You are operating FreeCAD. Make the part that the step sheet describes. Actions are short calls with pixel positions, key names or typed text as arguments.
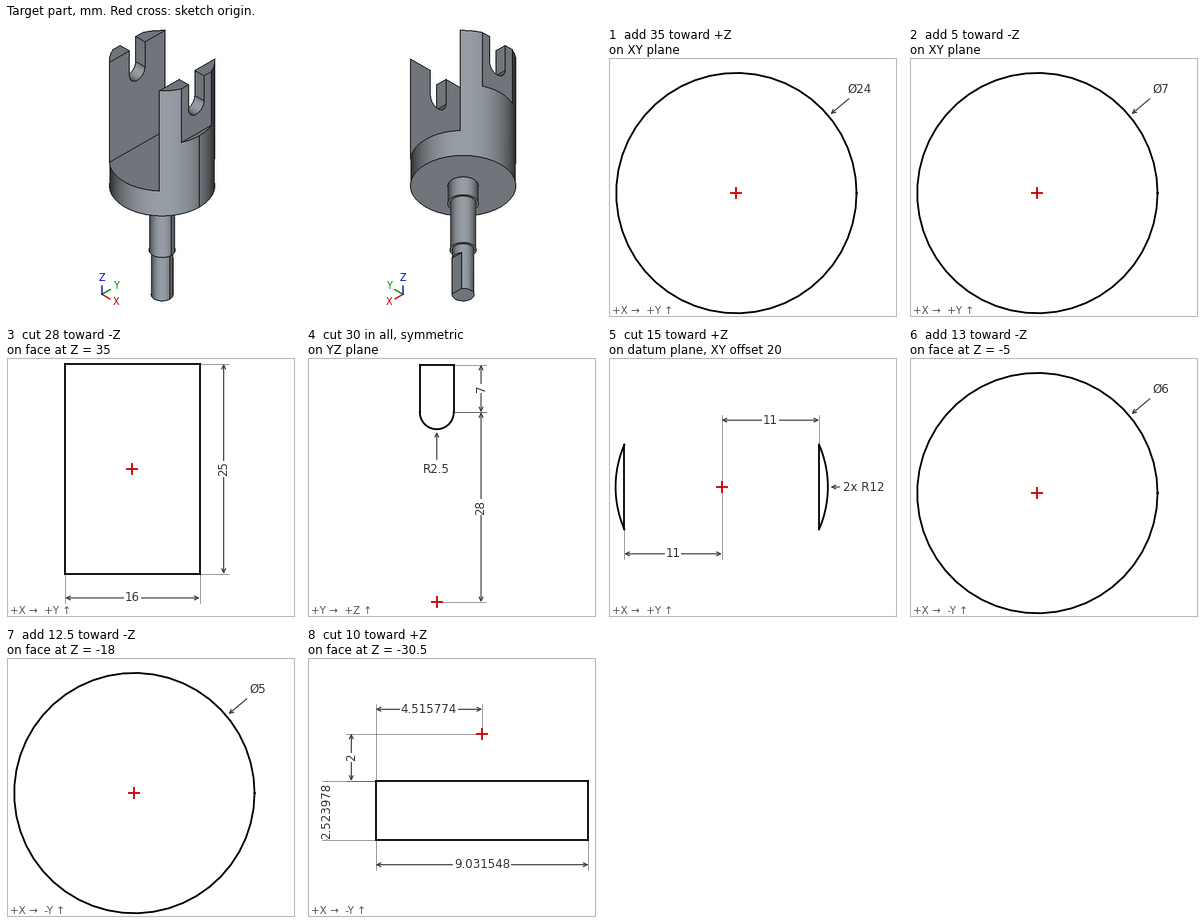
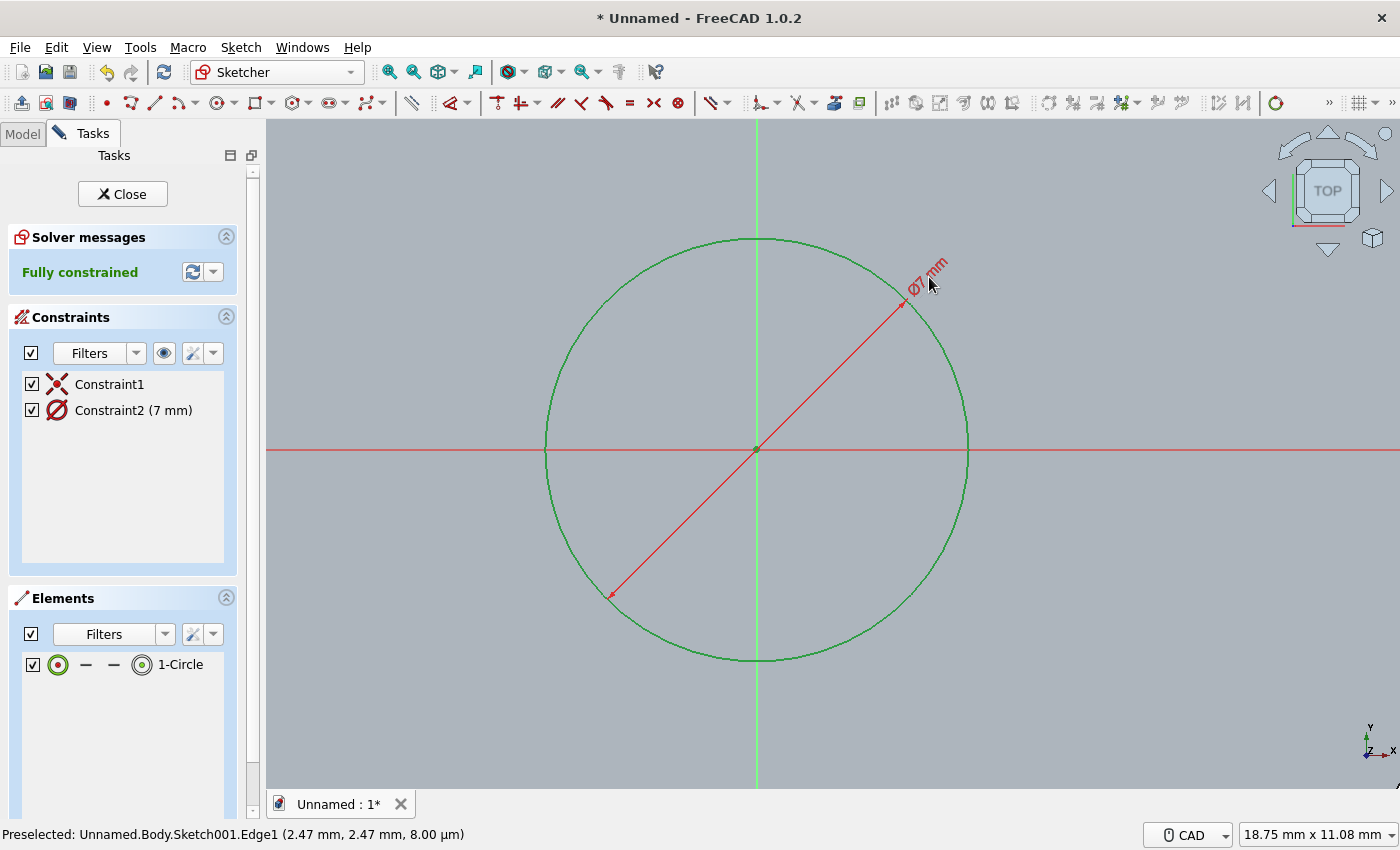
click(123, 194)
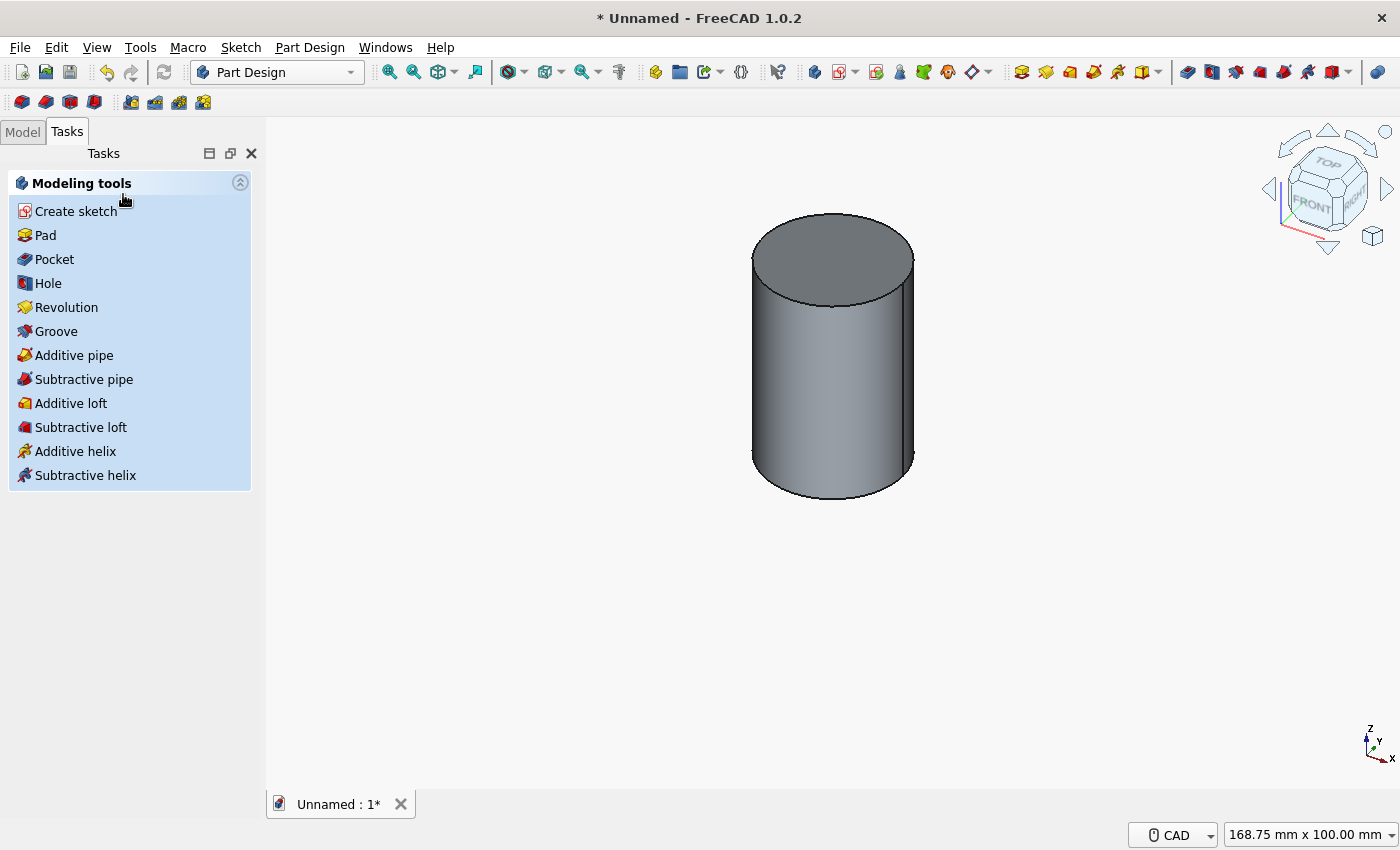
click(1022, 72)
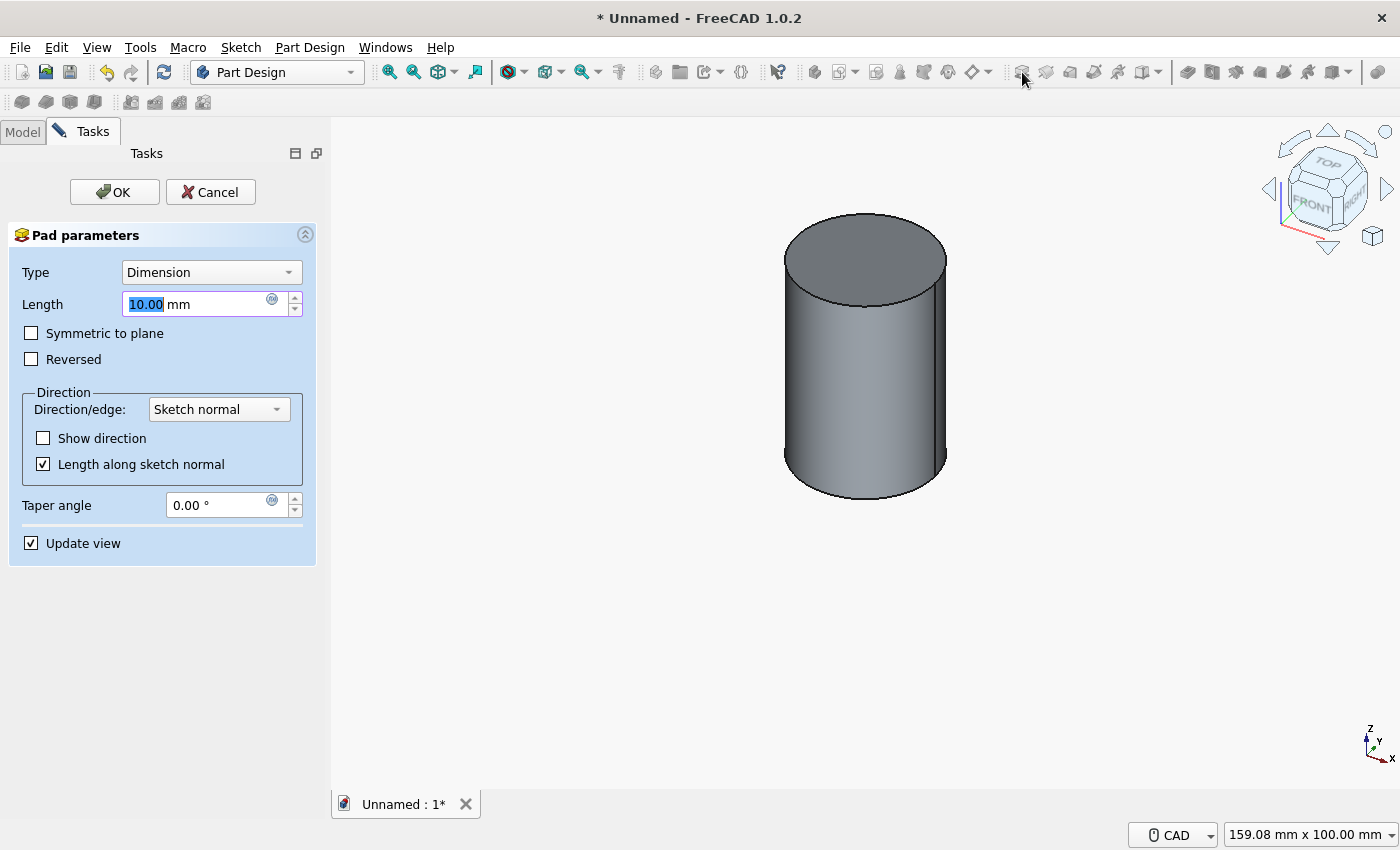
text(5)
key(Tab)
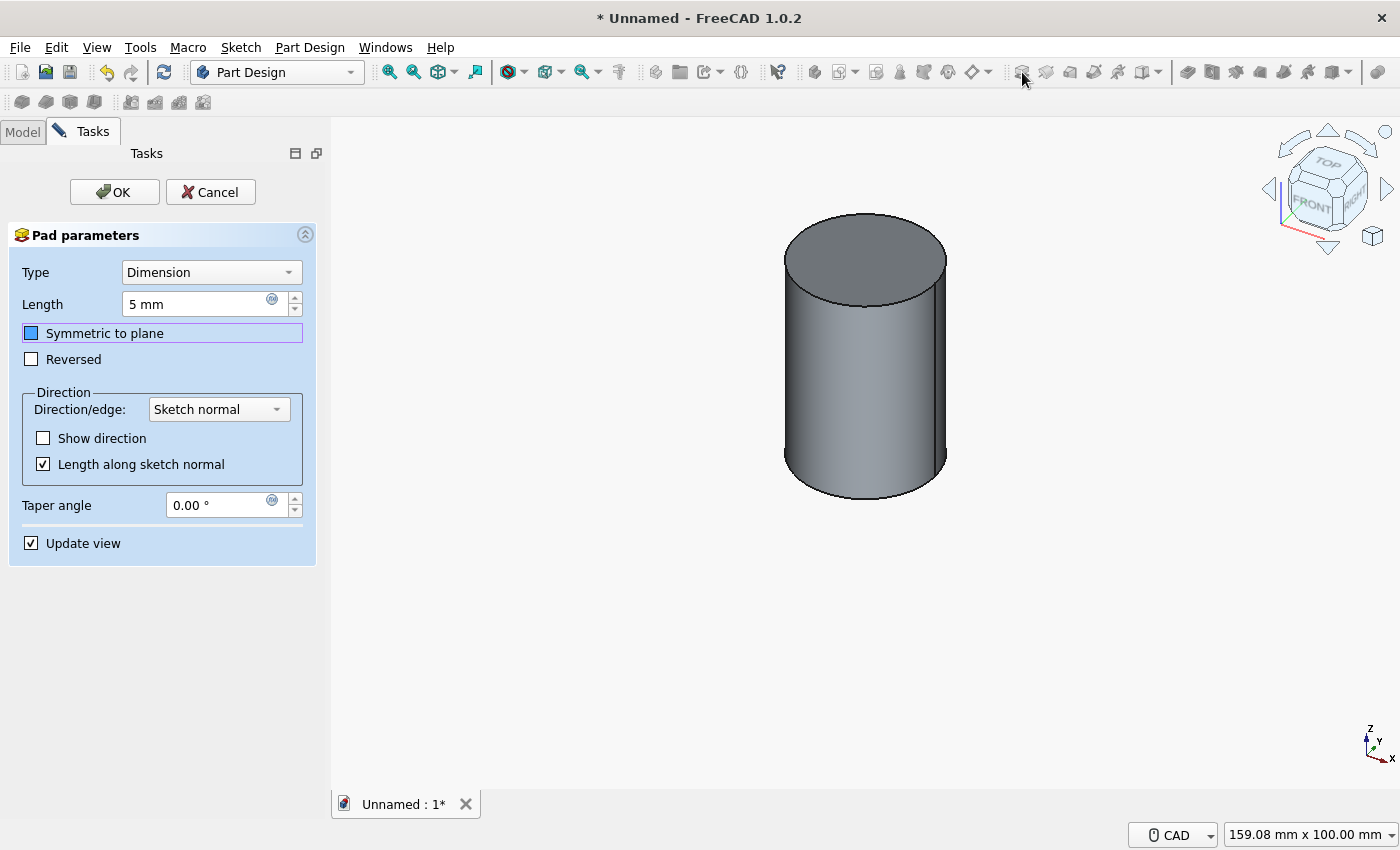
click(30, 359)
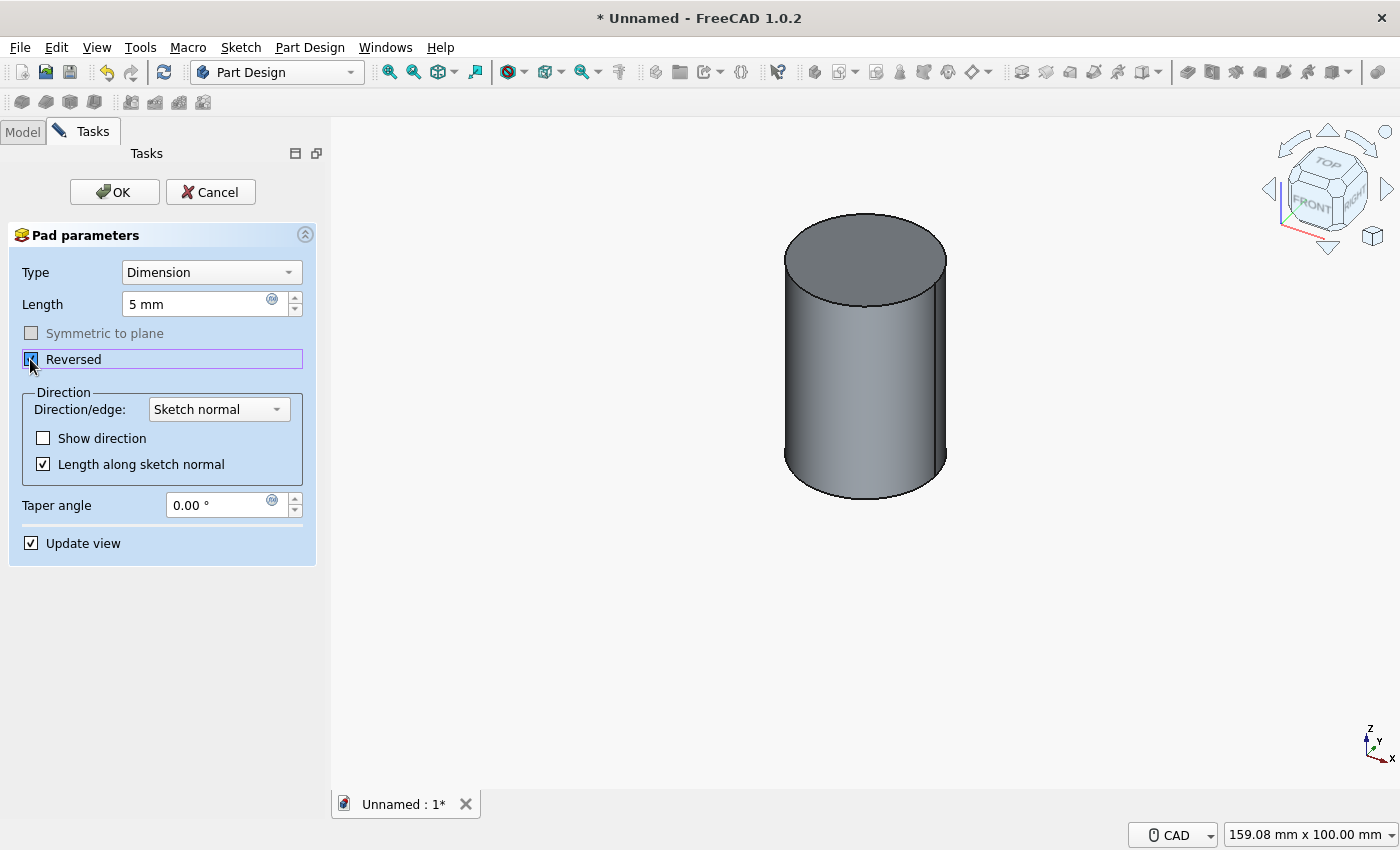
click(115, 192)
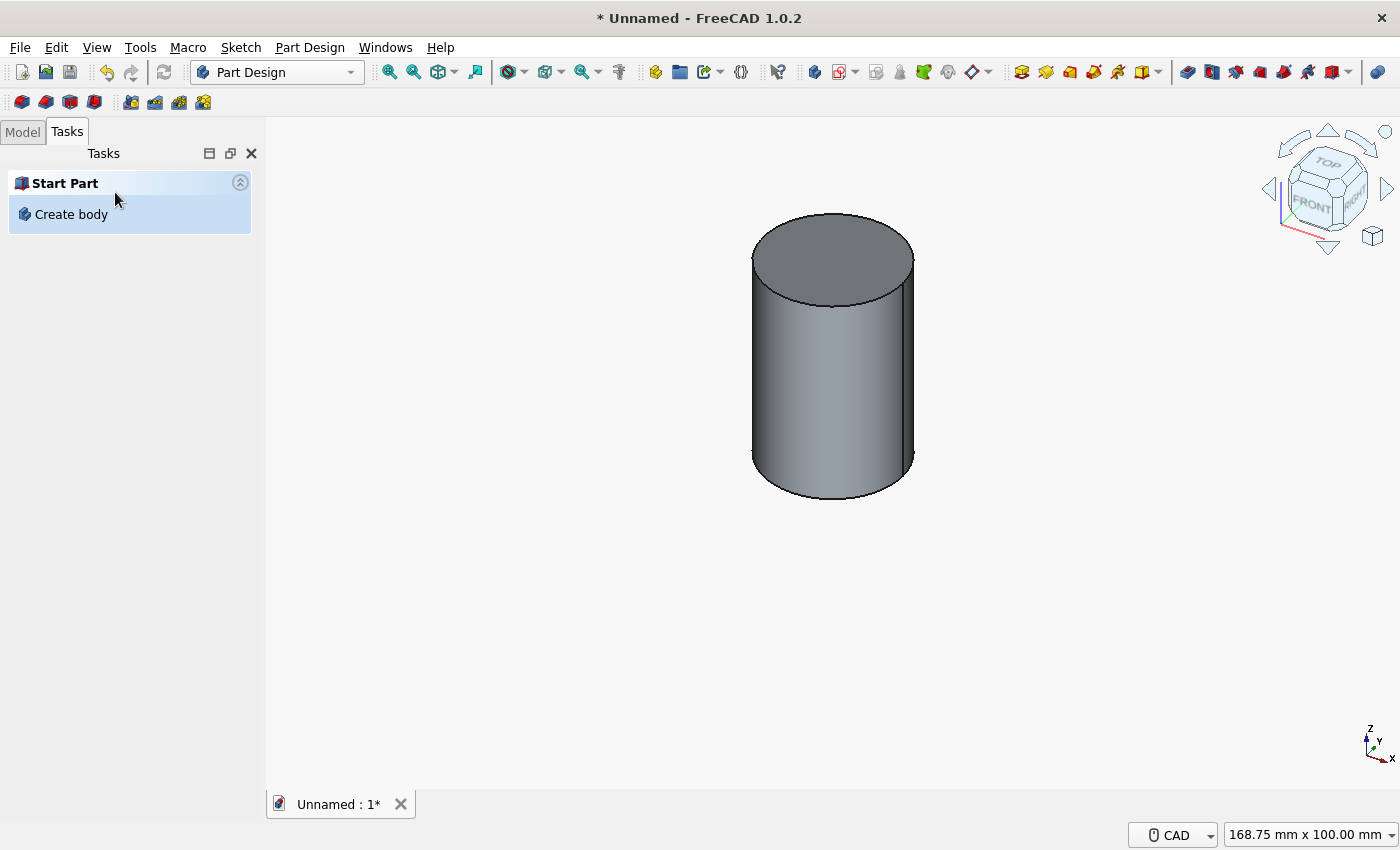
click(833, 259)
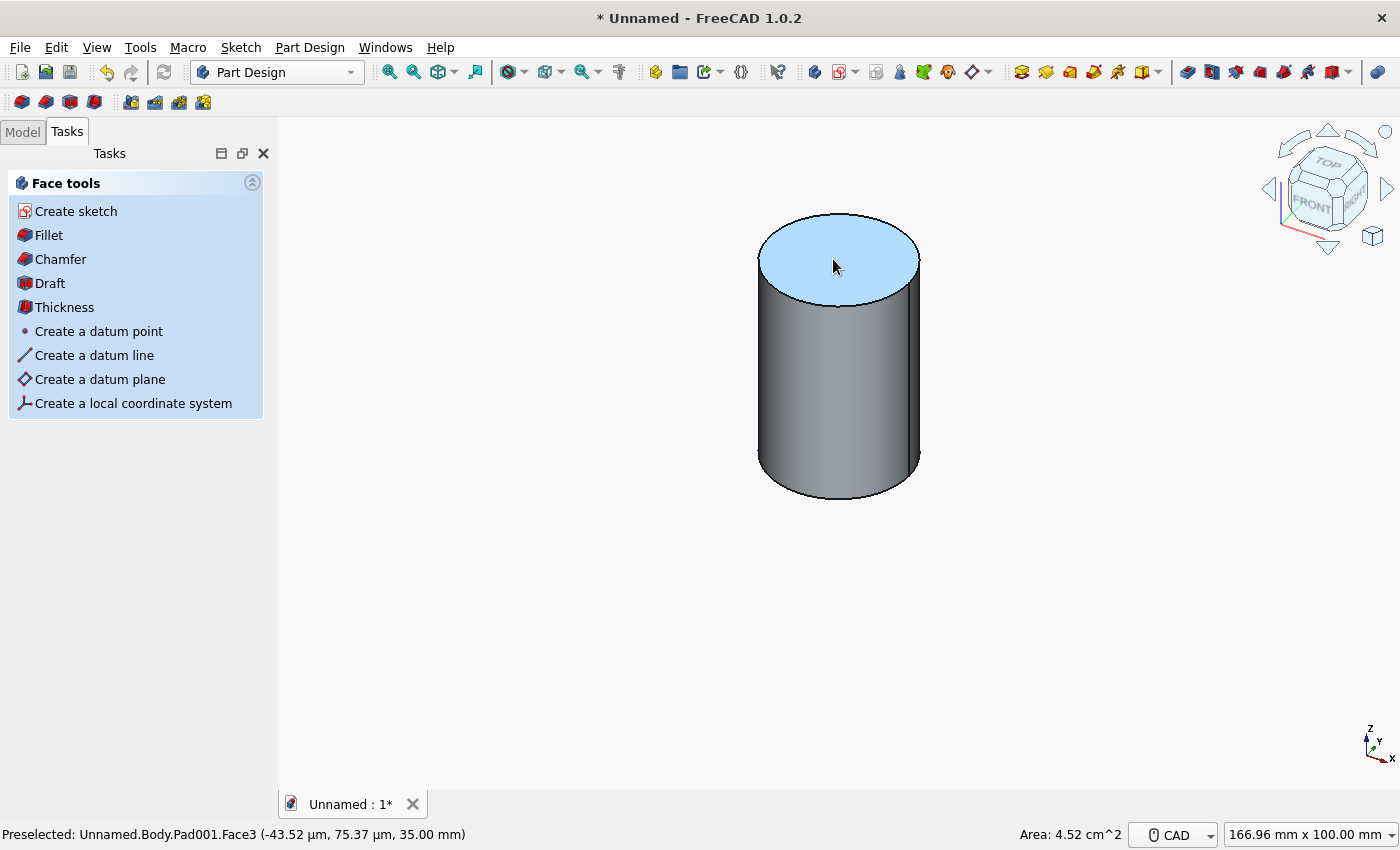
click(840, 72)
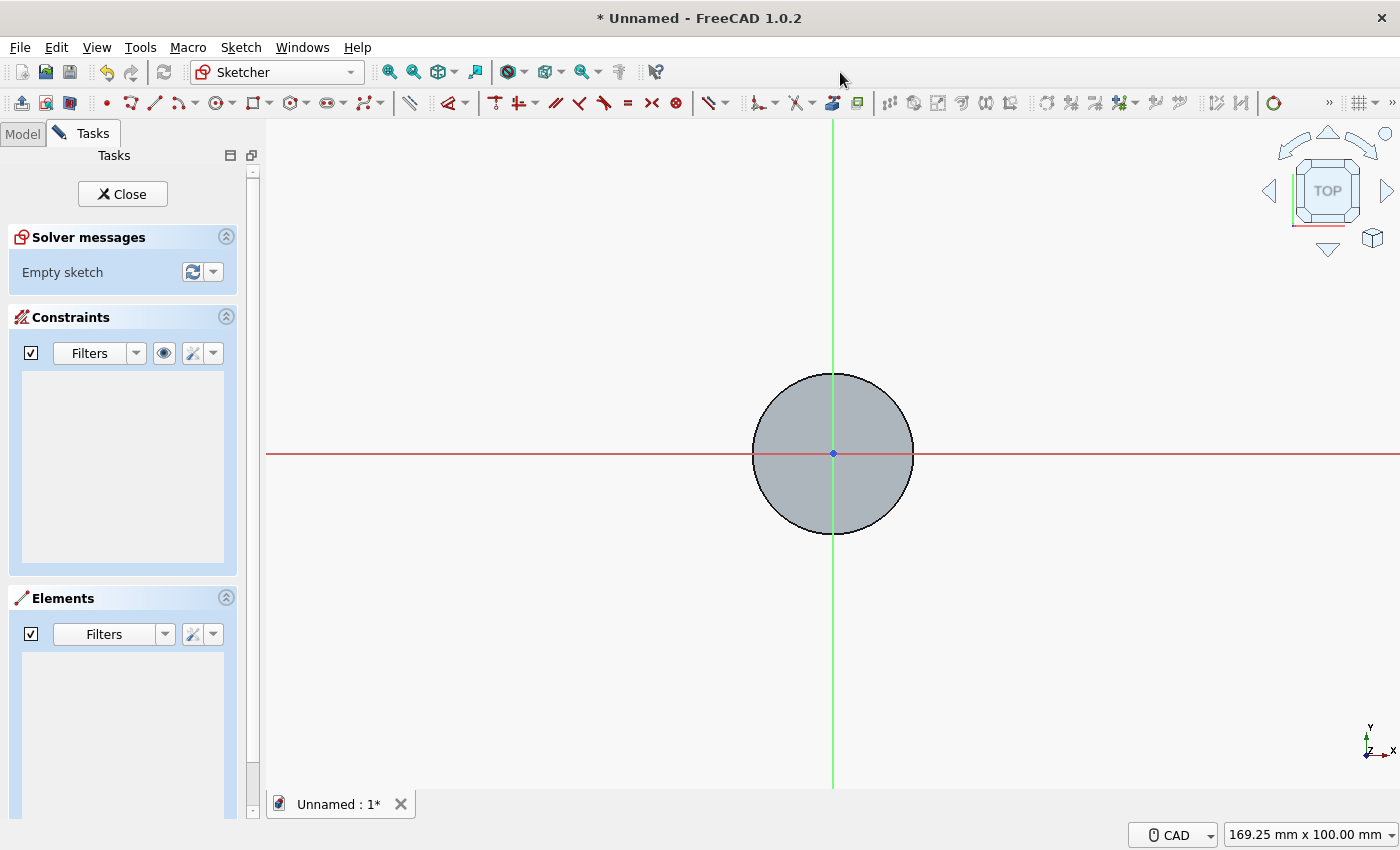
scroll(873, 454, up, 5)